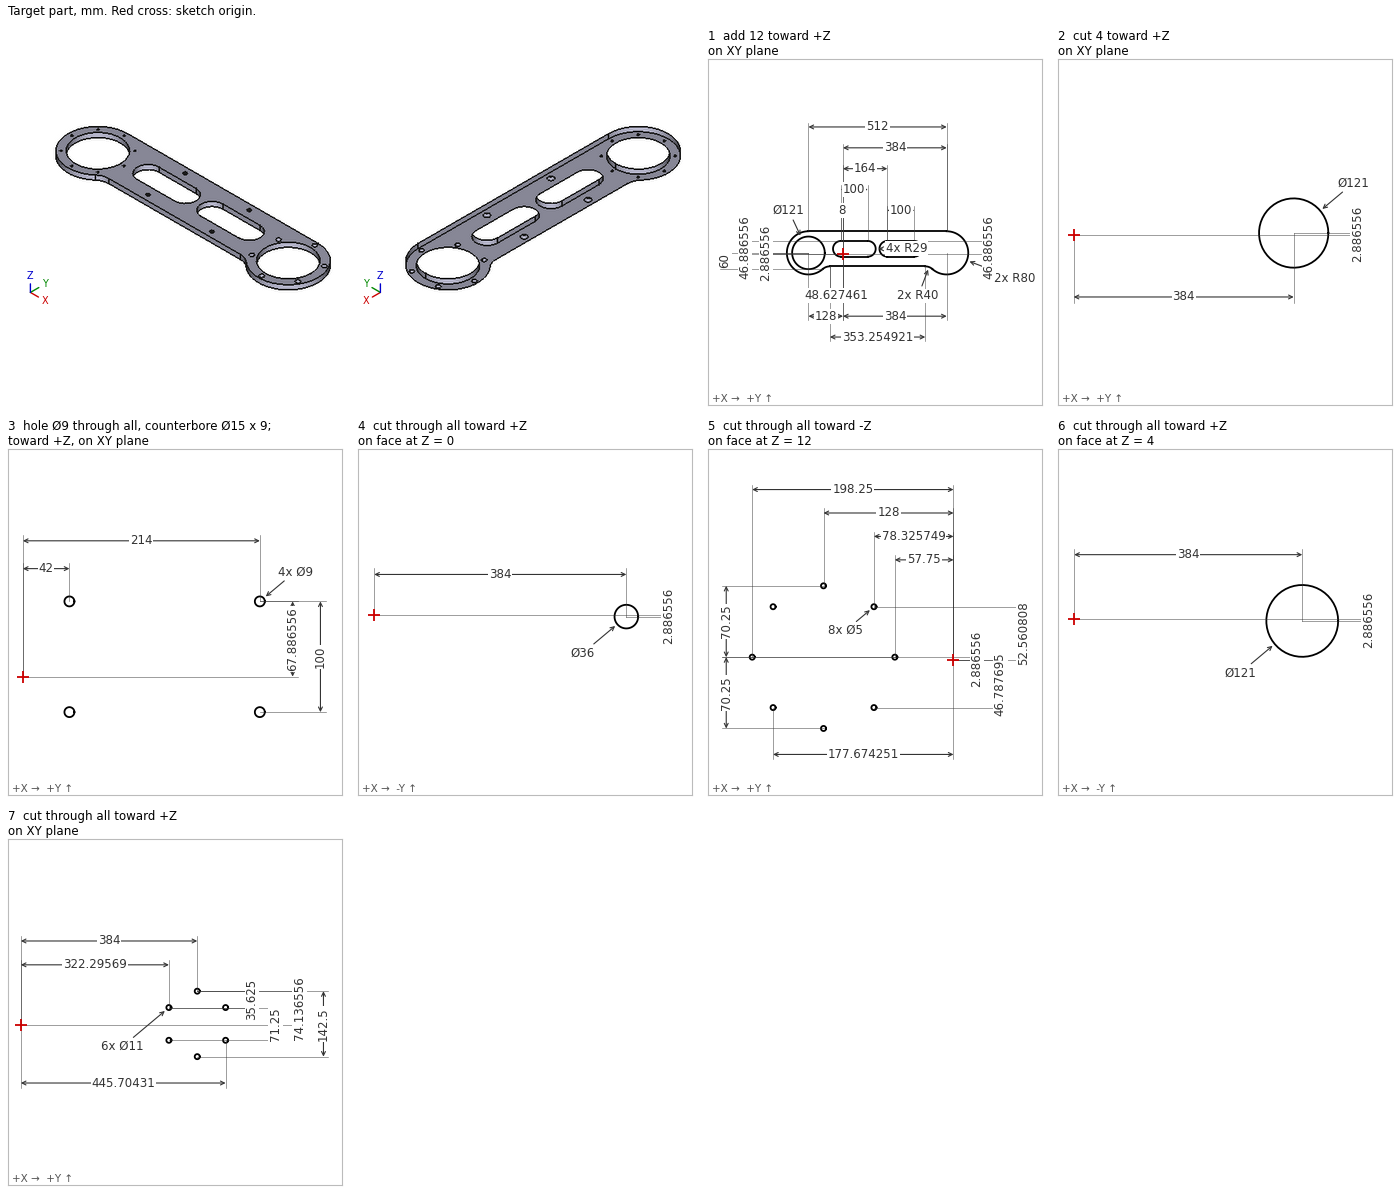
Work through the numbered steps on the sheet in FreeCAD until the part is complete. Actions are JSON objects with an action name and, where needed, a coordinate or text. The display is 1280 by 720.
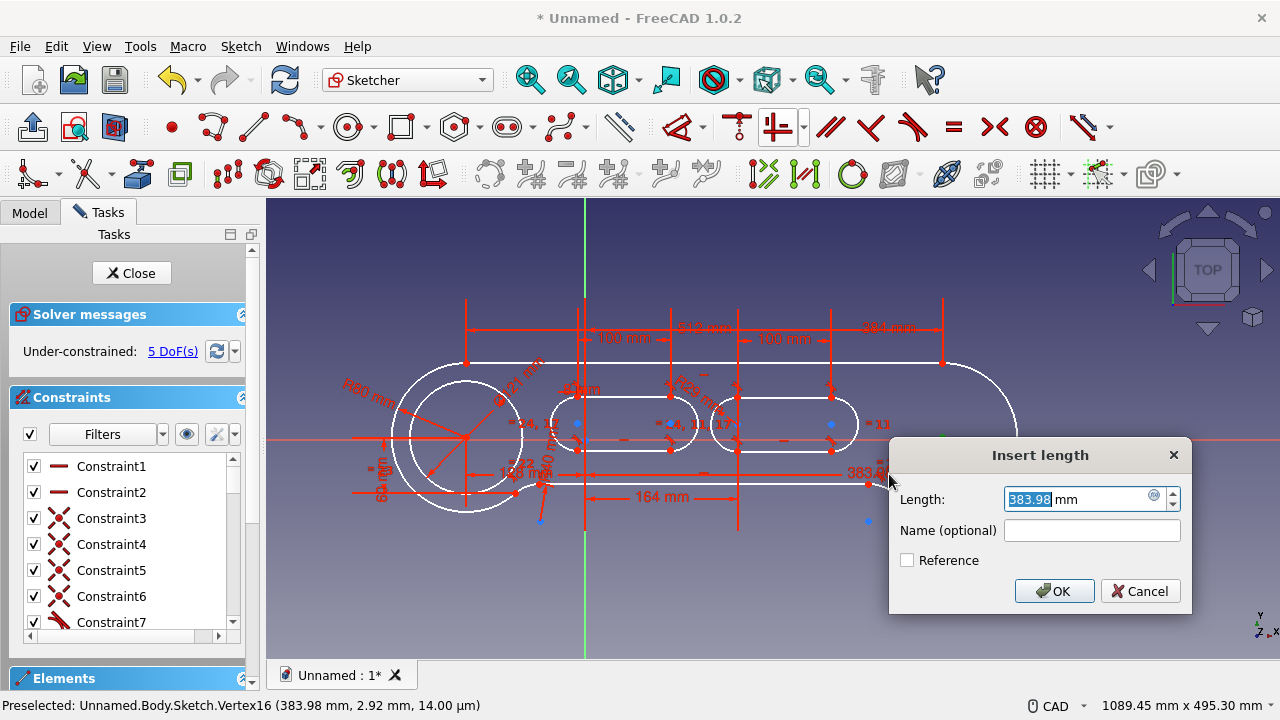
{"action": "type", "text": "384"}
{"action": "key", "text": "Return"}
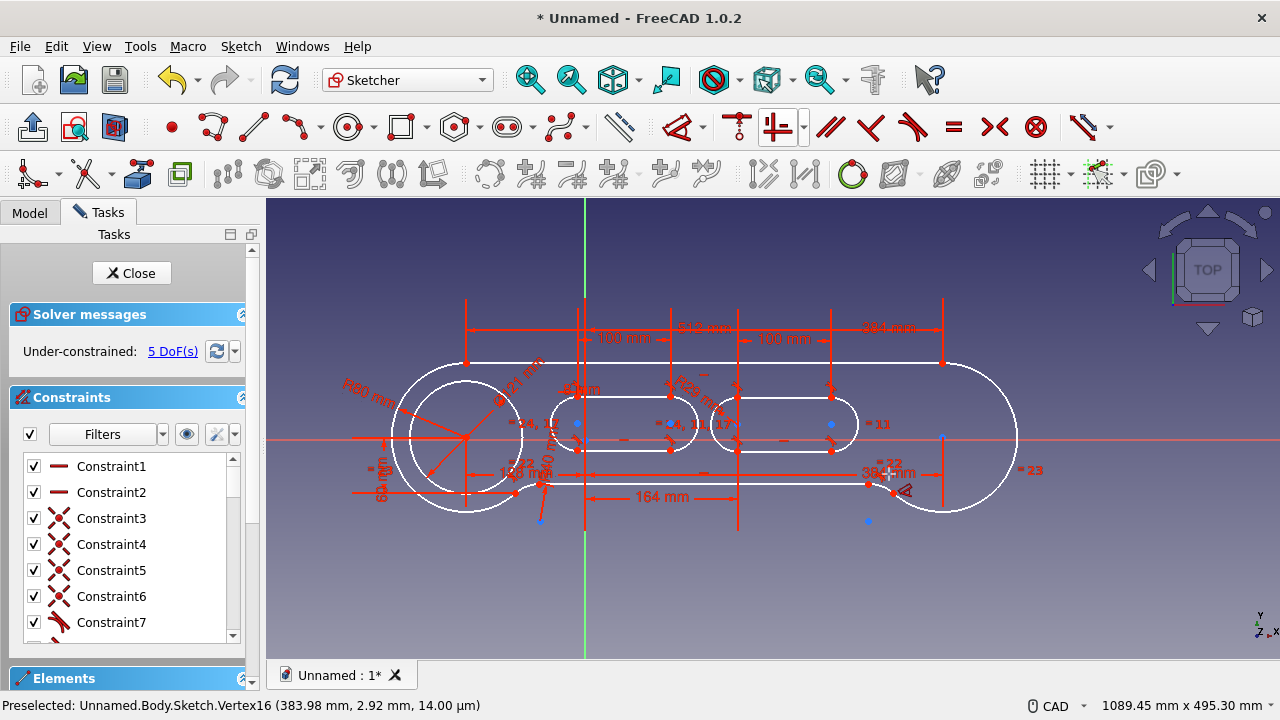
{"action": "scroll", "coordinate": [466, 438], "scroll_direction": "up", "scroll_amount": 14}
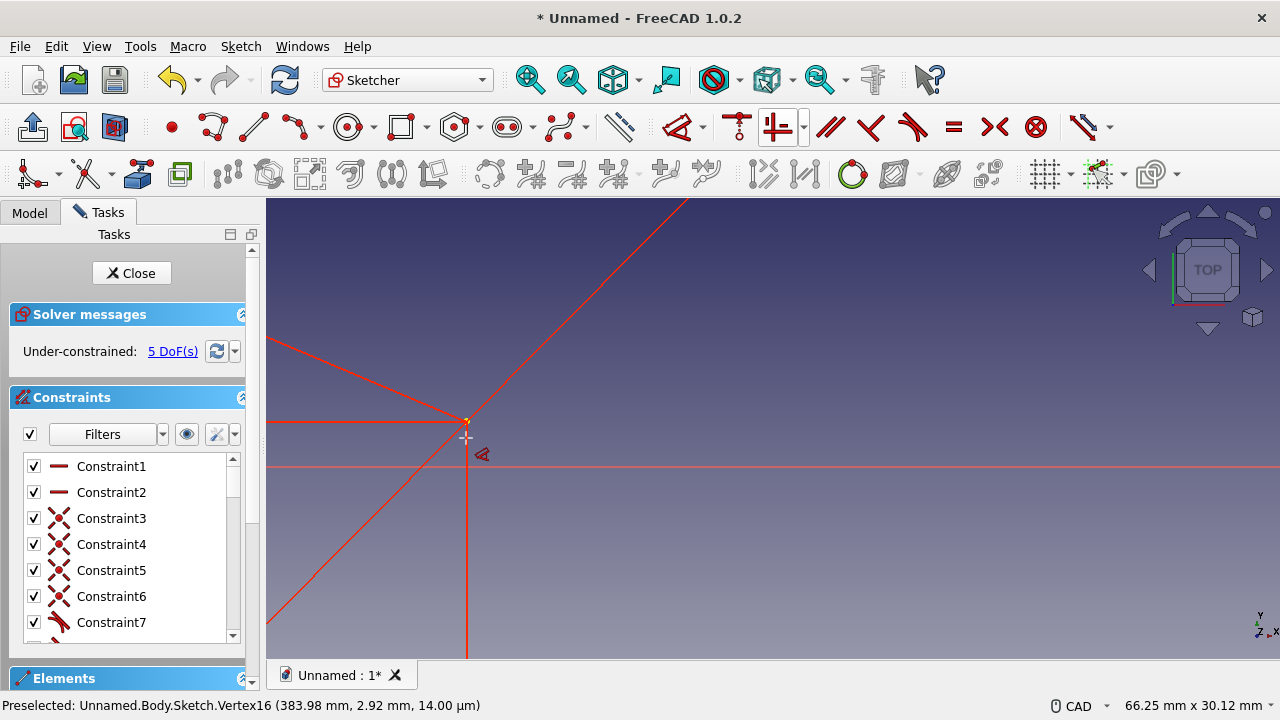
{"action": "left_click", "coordinate": [467, 422]}
{"action": "left_click", "coordinate": [433, 444]}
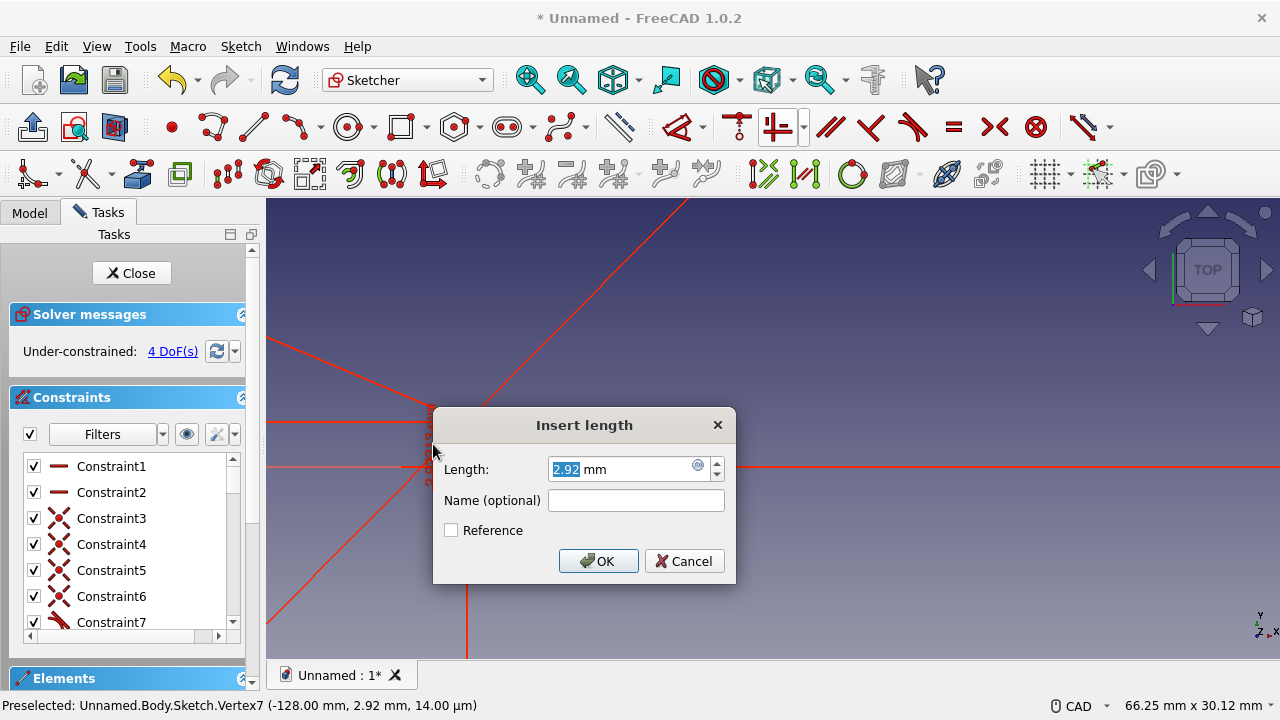
{"action": "type", "text": "2.886556"}
{"action": "key", "text": "Return"}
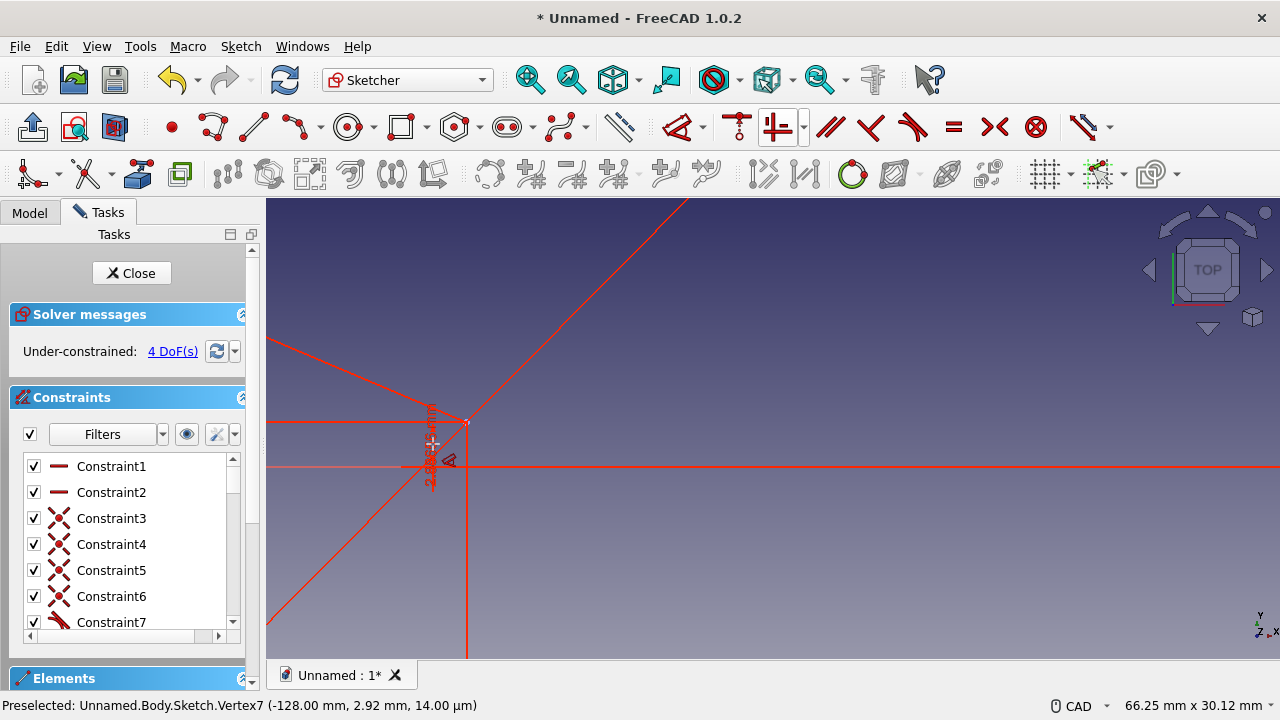
{"action": "scroll", "coordinate": [466, 439], "scroll_direction": "down", "scroll_amount": 14}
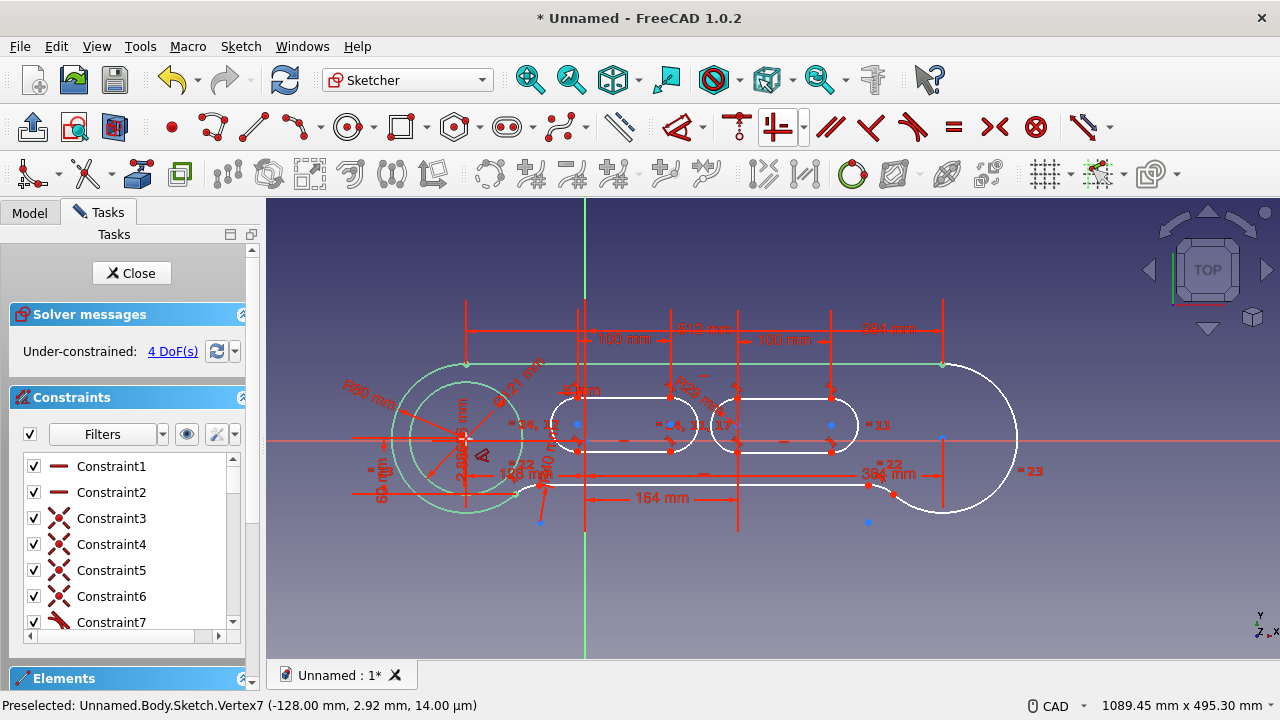
{"action": "left_click", "coordinate": [638, 485]}
{"action": "left_click", "coordinate": [780, 519]}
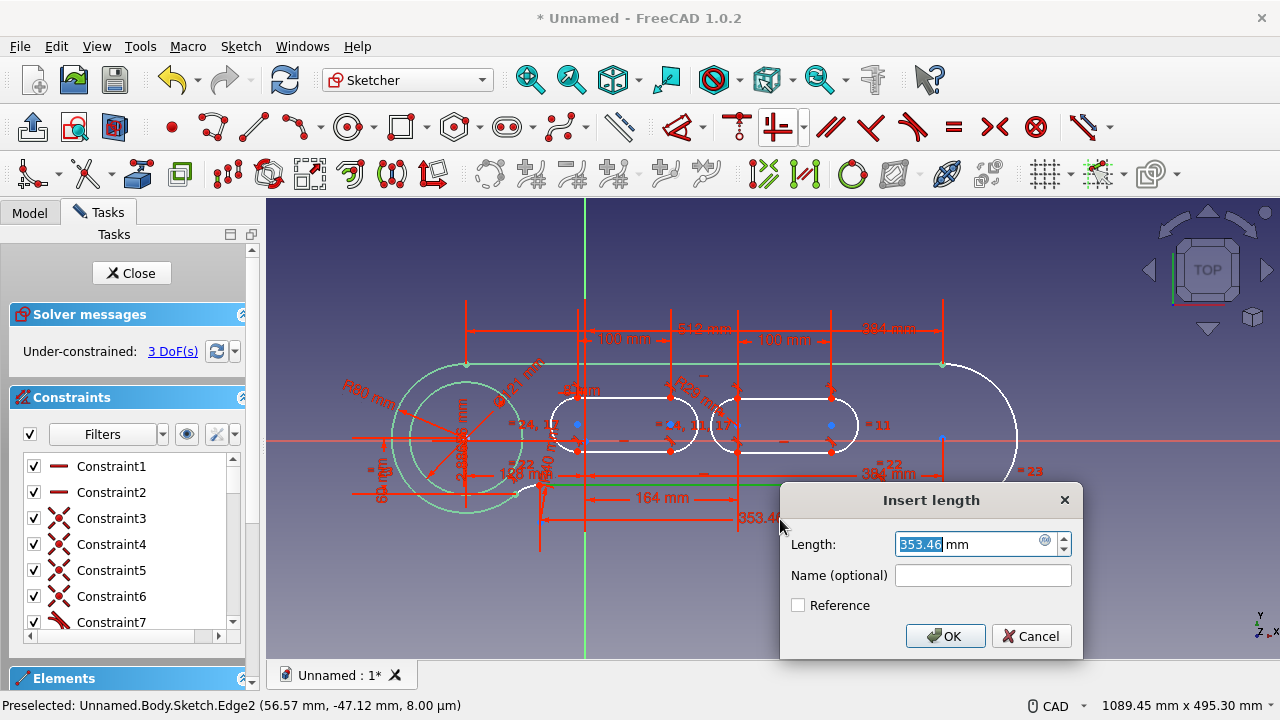
{"action": "type", "text": "353.254921"}
{"action": "key", "text": "Return"}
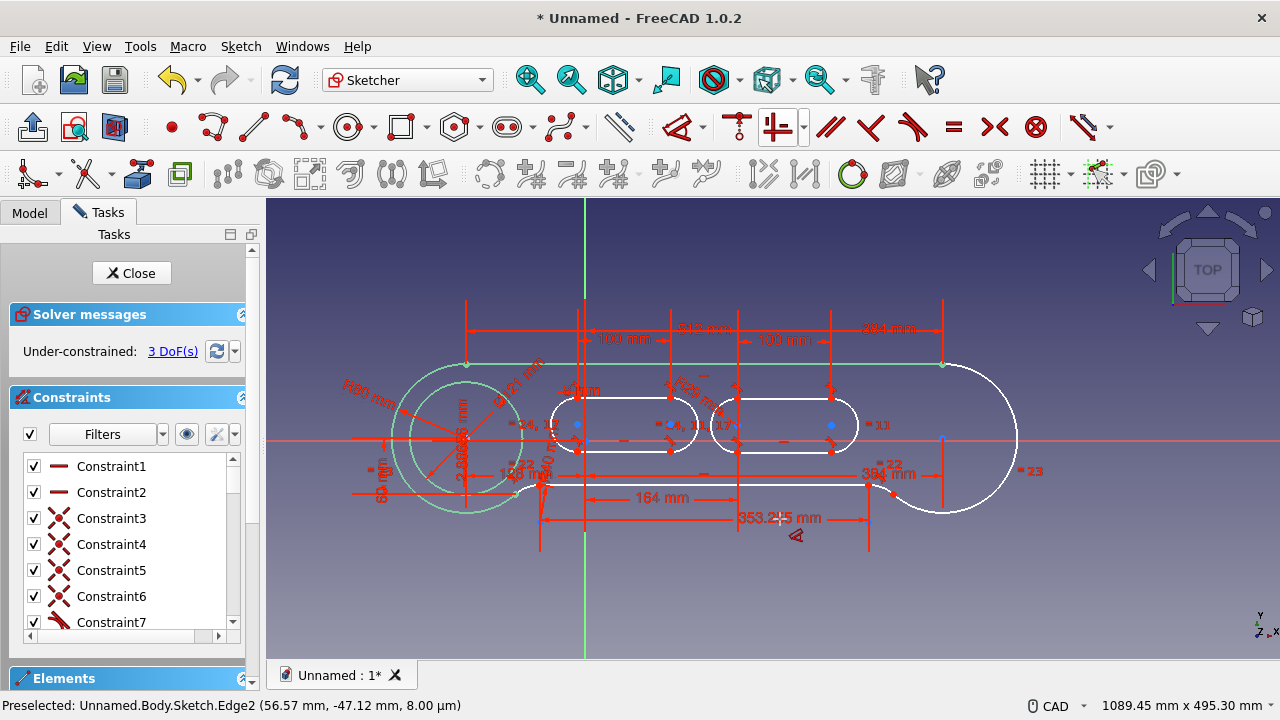
{"action": "left_click", "coordinate": [540, 485]}
{"action": "left_click", "coordinate": [563, 519]}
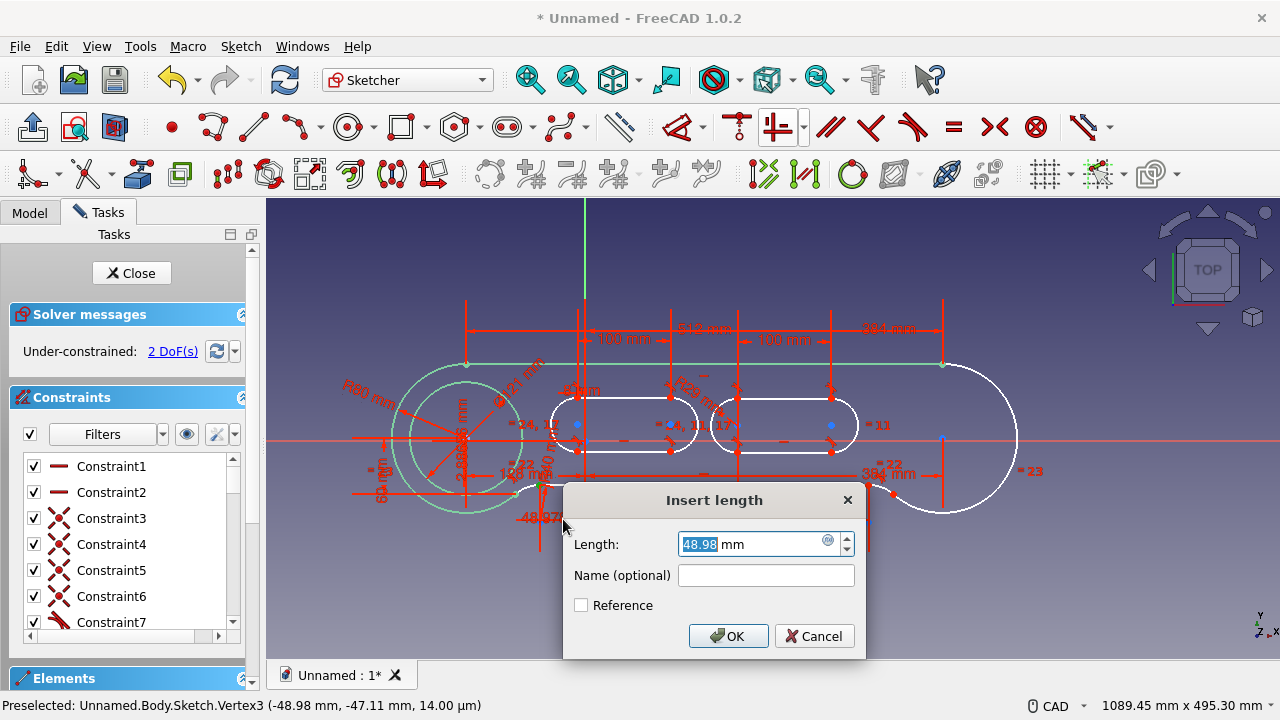
{"action": "type", "text": "48.627461"}
{"action": "key", "text": "Return"}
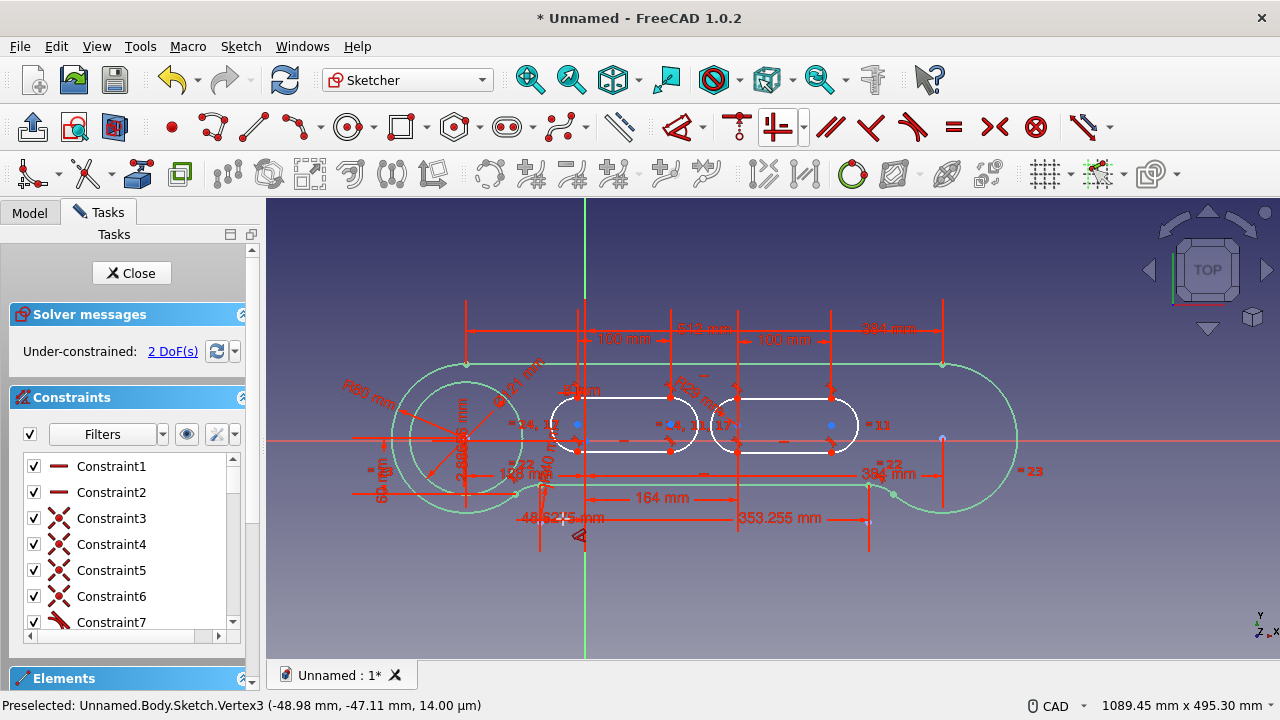
{"action": "left_click", "coordinate": [738, 399]}
{"action": "left_click", "coordinate": [772, 420]}